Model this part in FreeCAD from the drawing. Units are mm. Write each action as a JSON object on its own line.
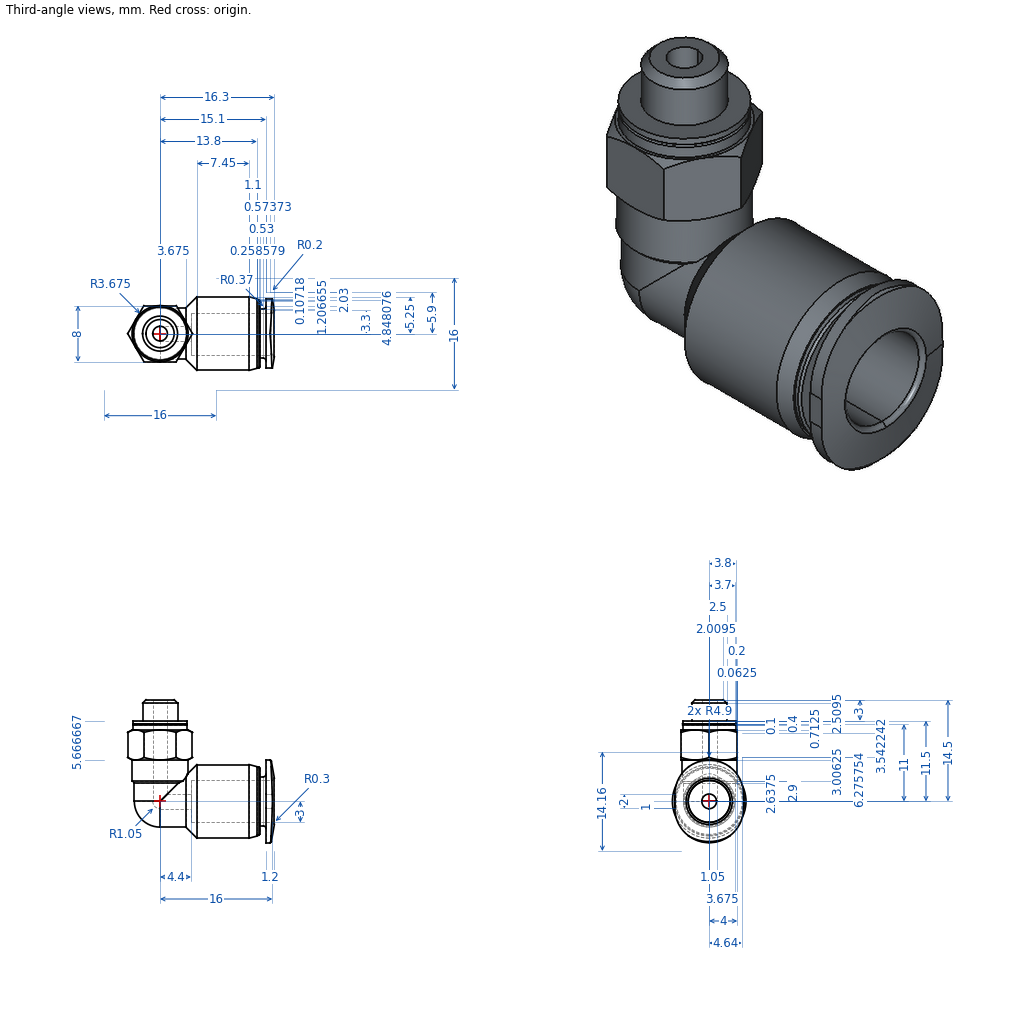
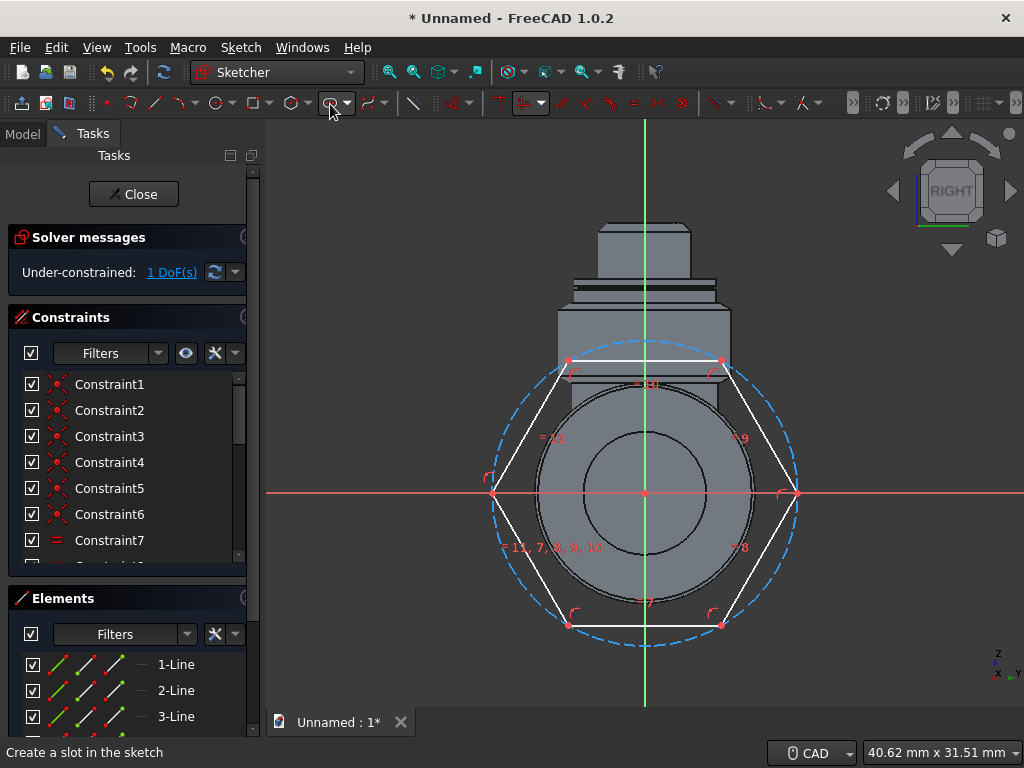
{"action": "left_click", "coordinate": [645, 512]}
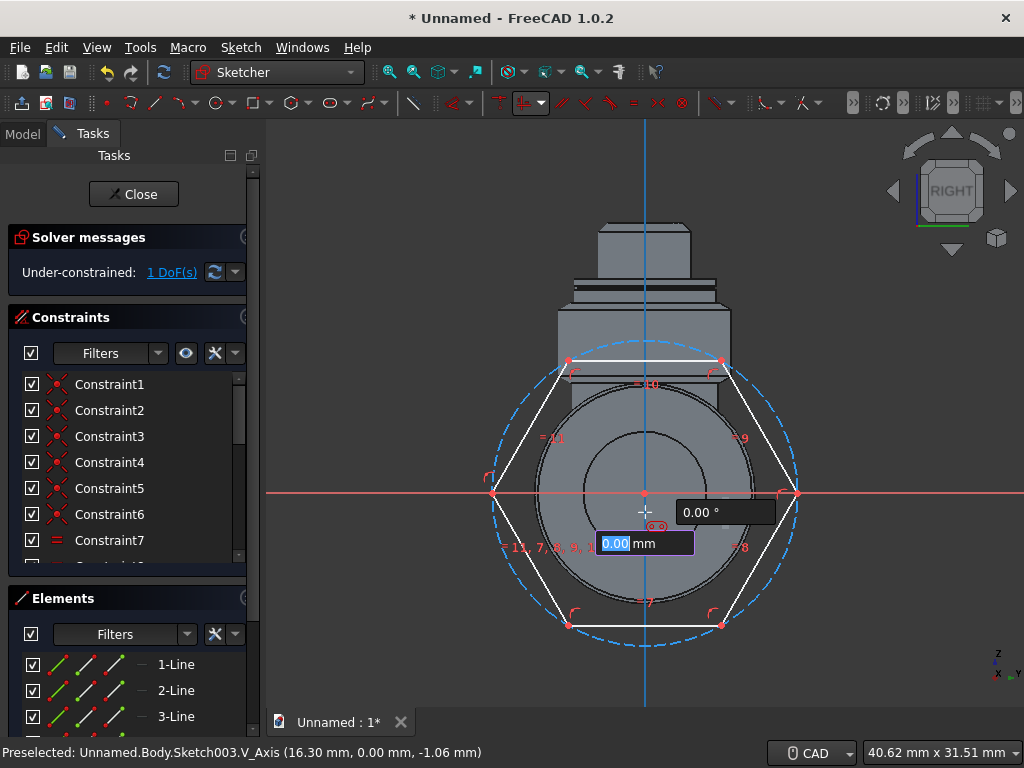
{"action": "left_click", "coordinate": [654, 475]}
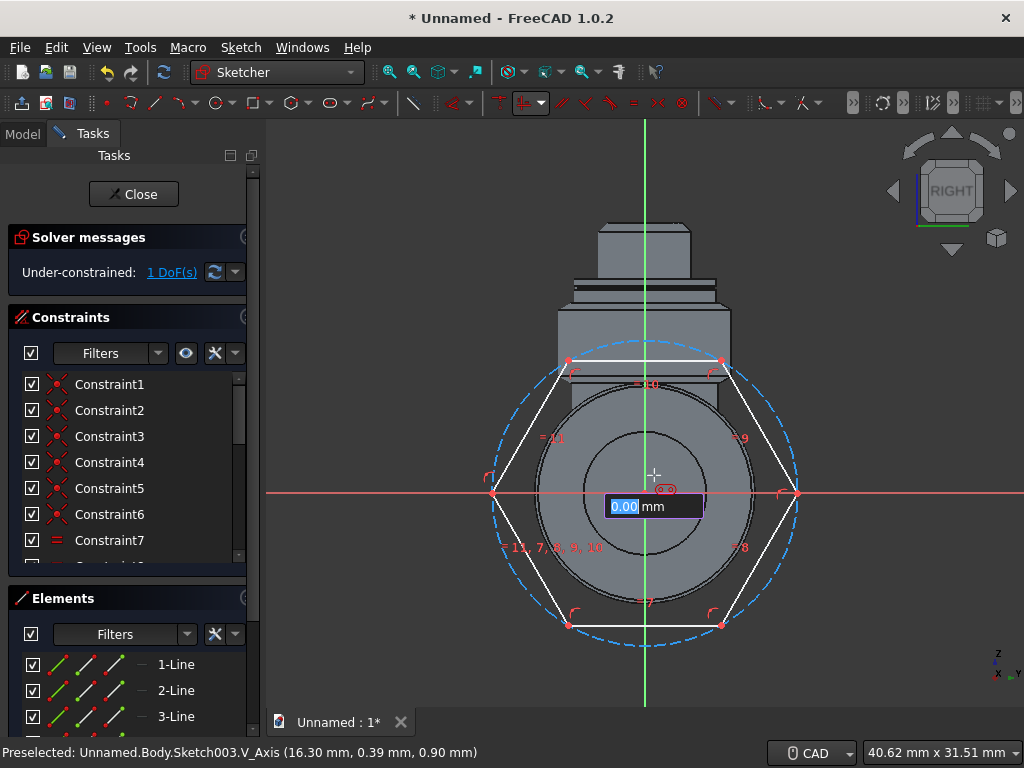
{"action": "scroll", "coordinate": [553, 499], "scroll_direction": "up", "scroll_amount": 6}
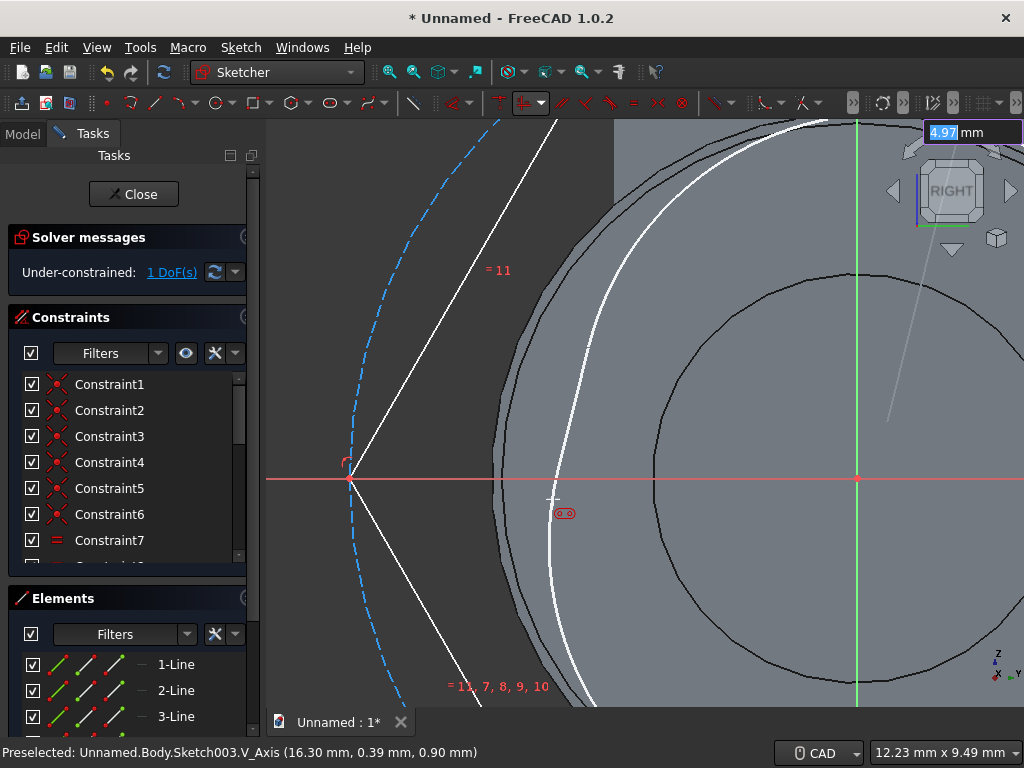
{"action": "left_click", "coordinate": [553, 497]}
{"action": "key", "text": "Escape"}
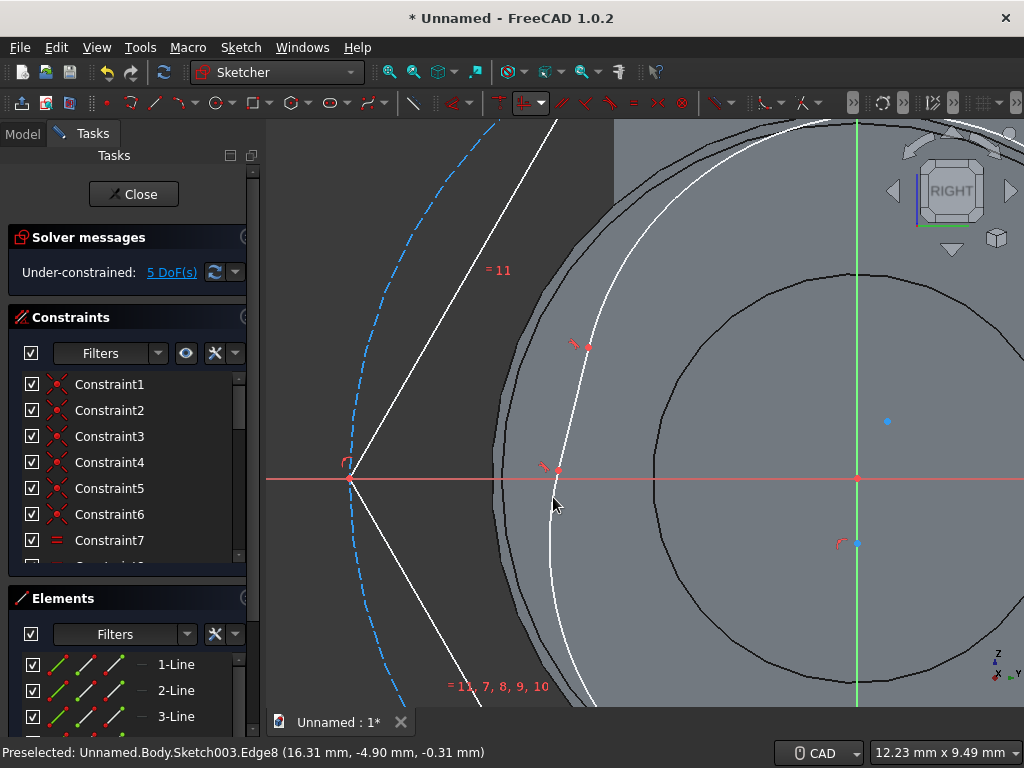
{"action": "scroll", "coordinate": [413, 375], "scroll_direction": "down", "scroll_amount": 5}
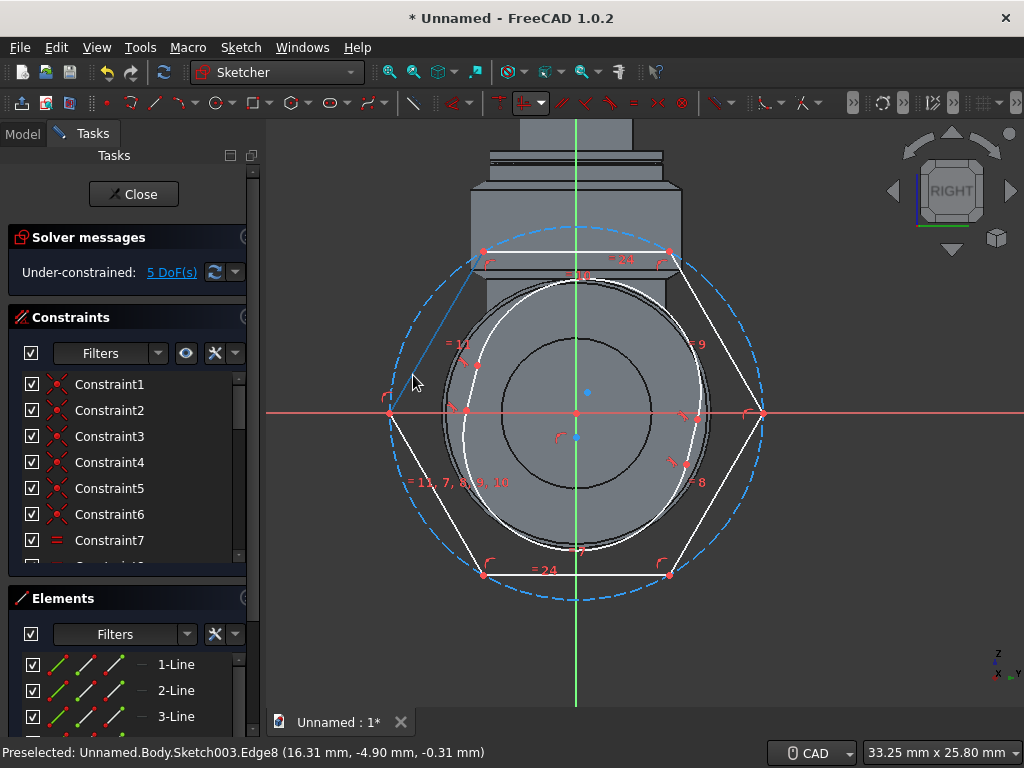
{"action": "left_click", "coordinate": [588, 392]}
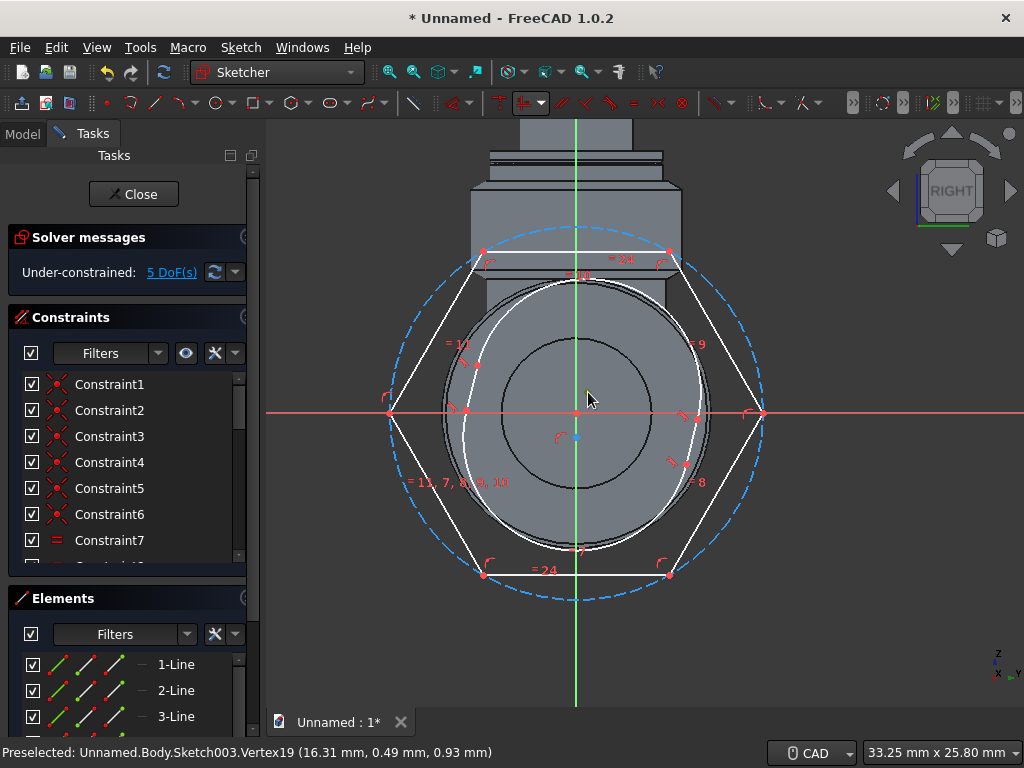
{"action": "left_click", "coordinate": [576, 641]}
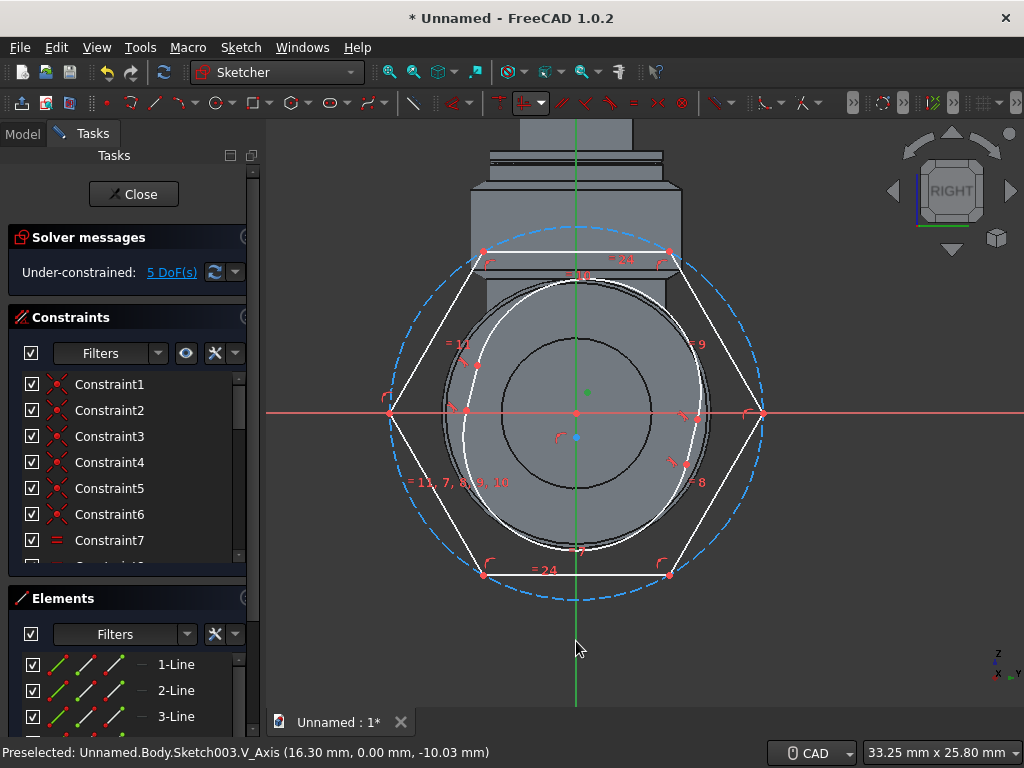
{"action": "left_click", "coordinate": [500, 104]}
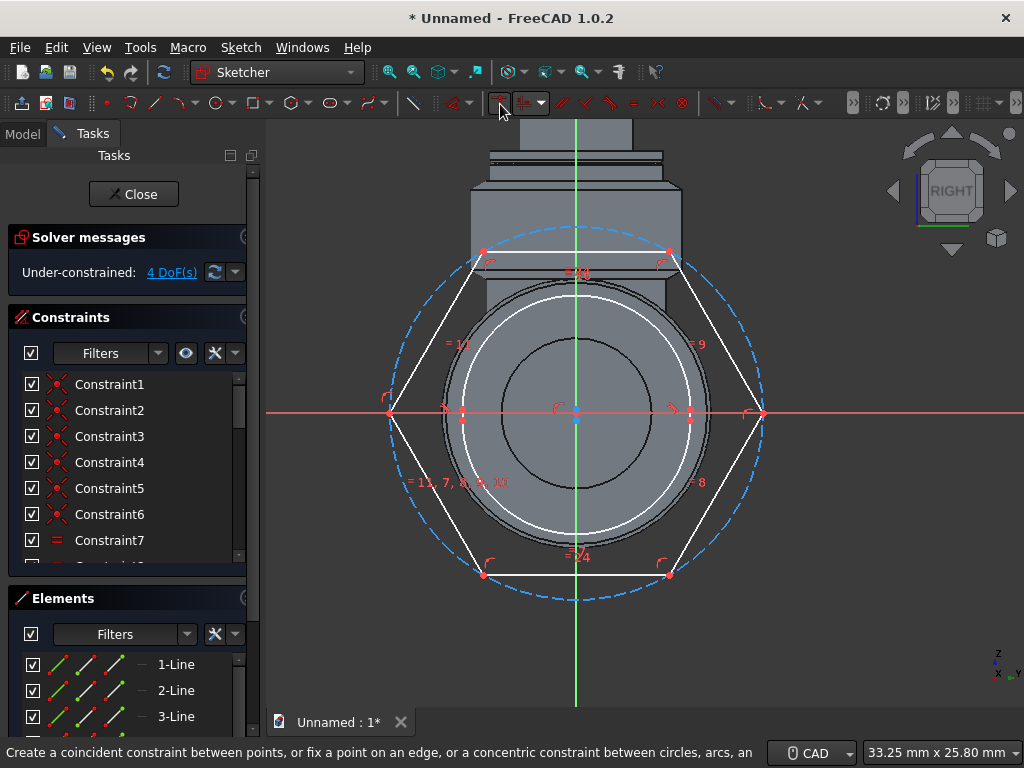
{"action": "left_click", "coordinate": [452, 104]}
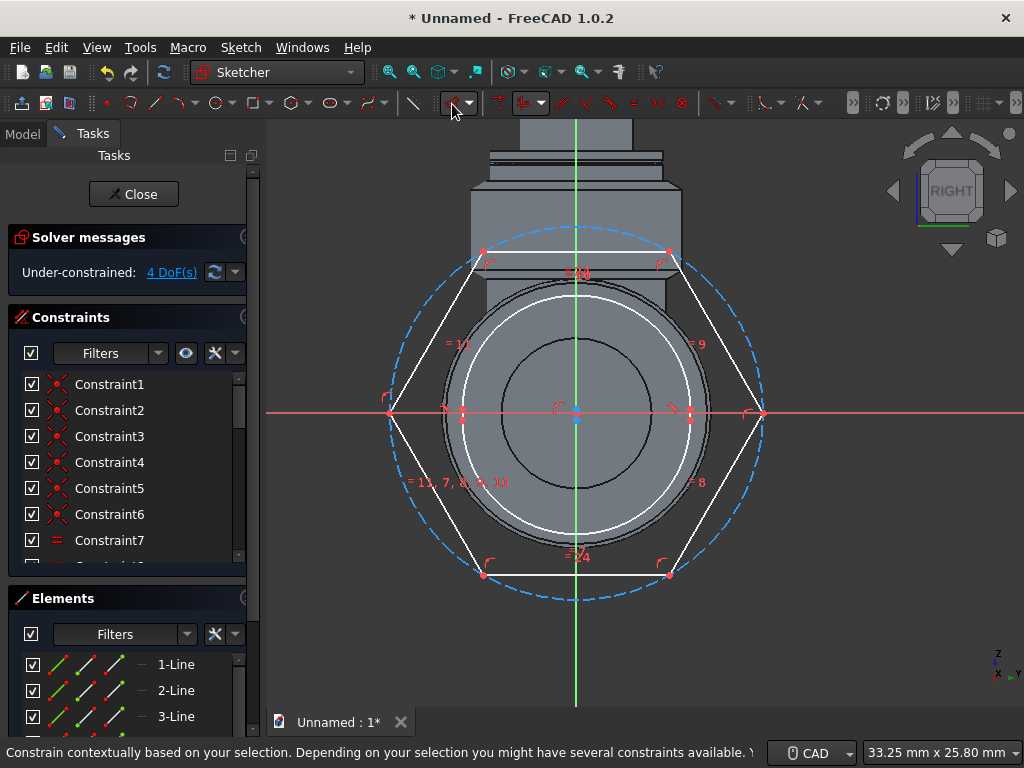
{"action": "left_click", "coordinate": [510, 512]}
{"action": "left_click", "coordinate": [491, 538]}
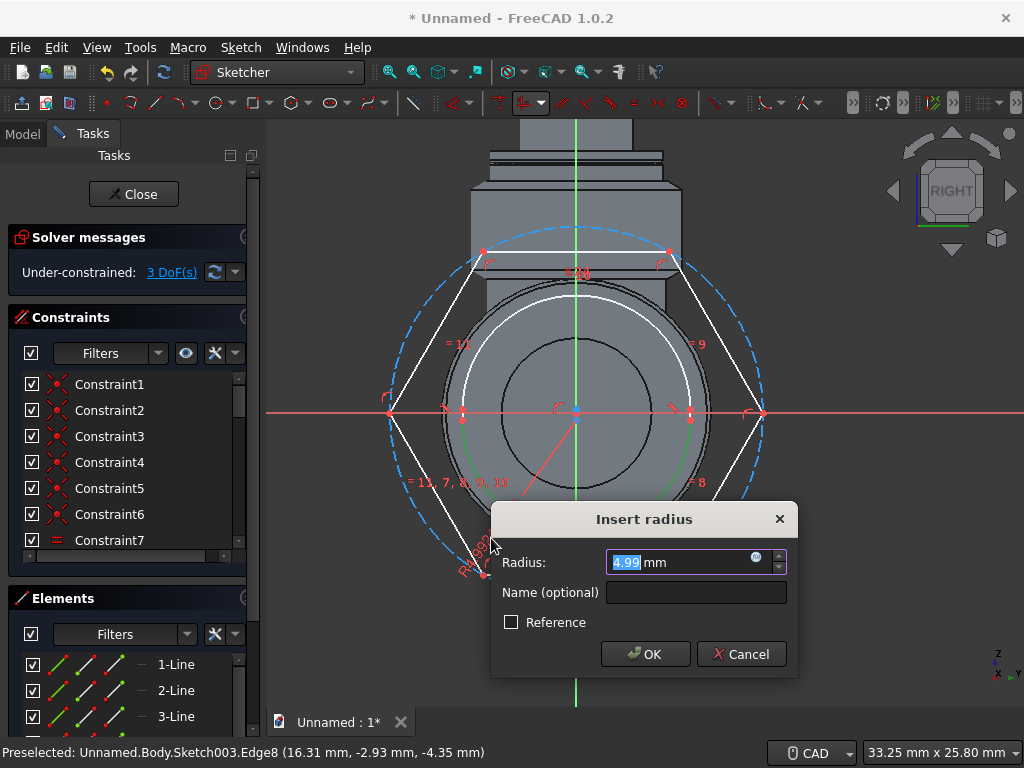
{"action": "type", "text": "4.9"}
{"action": "key", "text": "Return"}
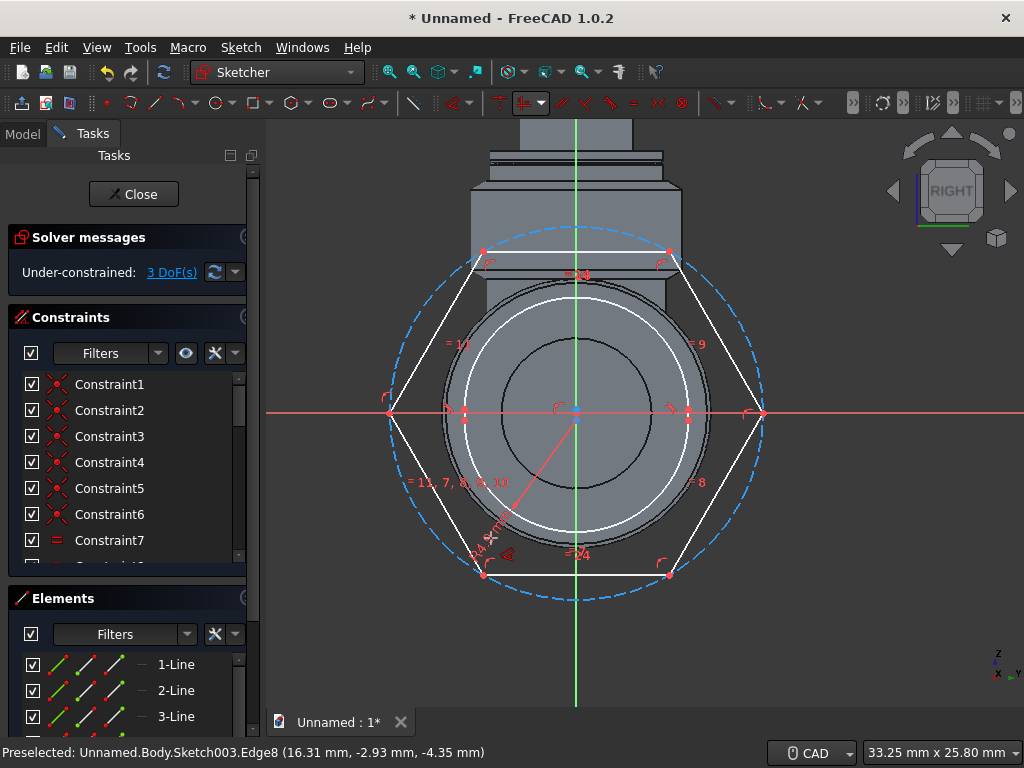
{"action": "scroll", "coordinate": [465, 415], "scroll_direction": "up", "scroll_amount": 5}